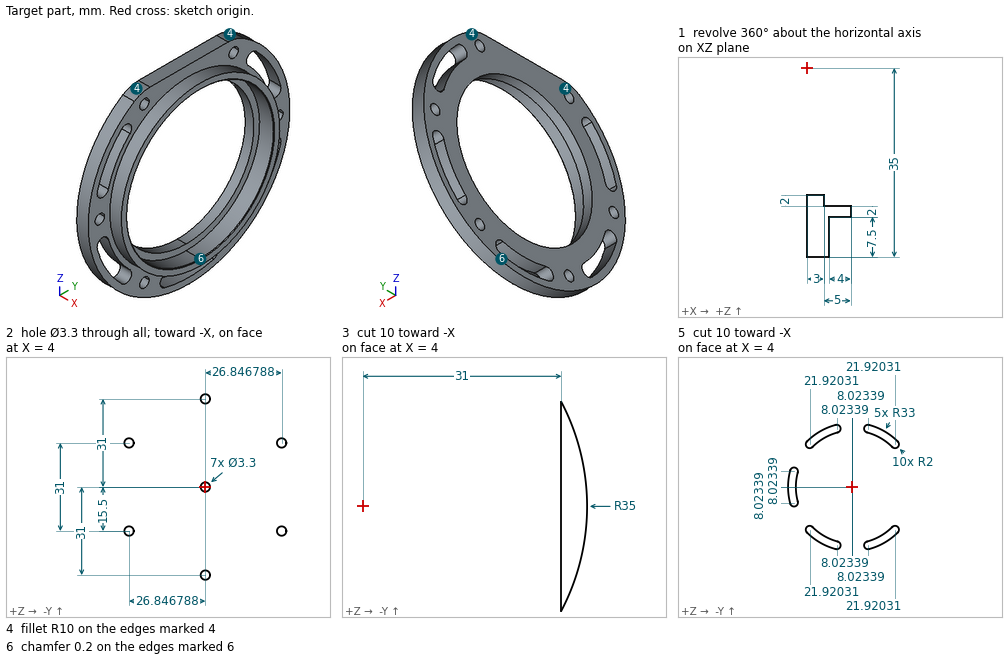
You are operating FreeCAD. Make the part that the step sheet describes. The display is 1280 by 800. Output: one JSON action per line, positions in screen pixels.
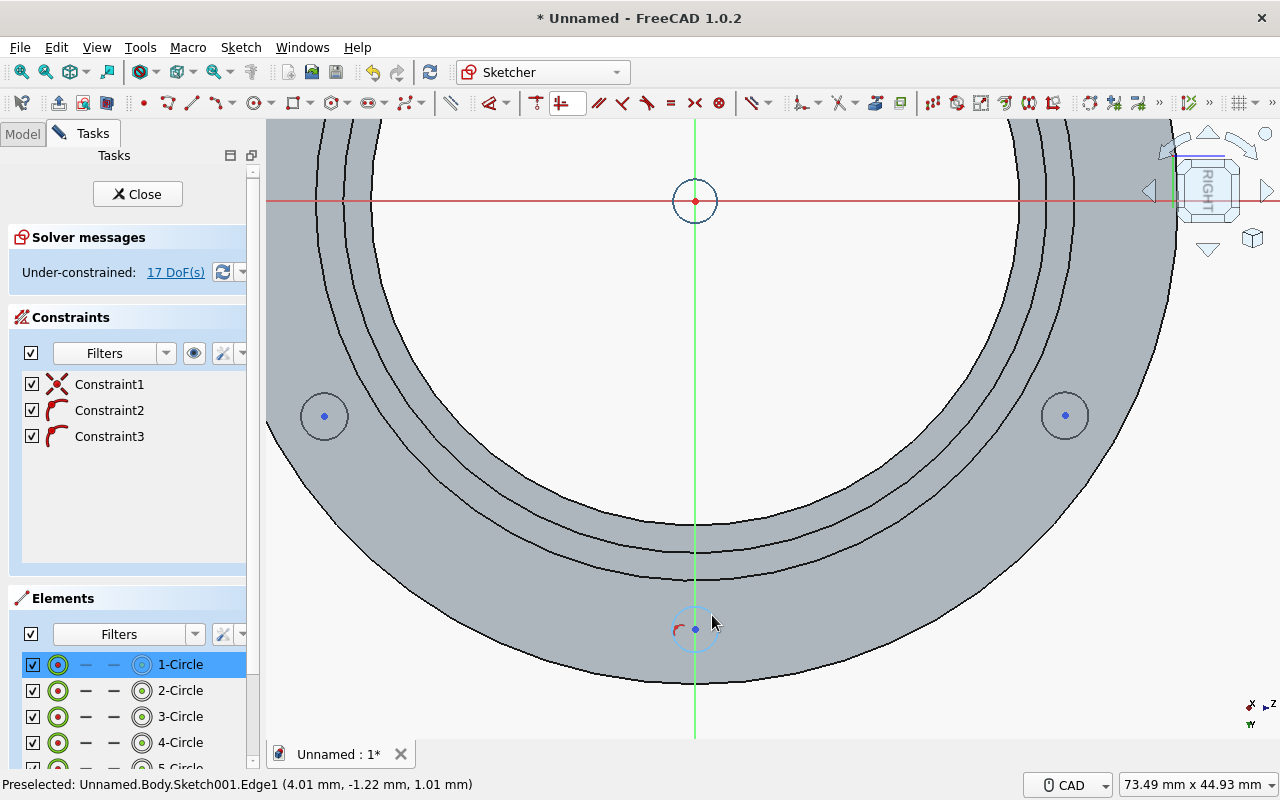
{"action": "left_click", "coordinate": [711, 613]}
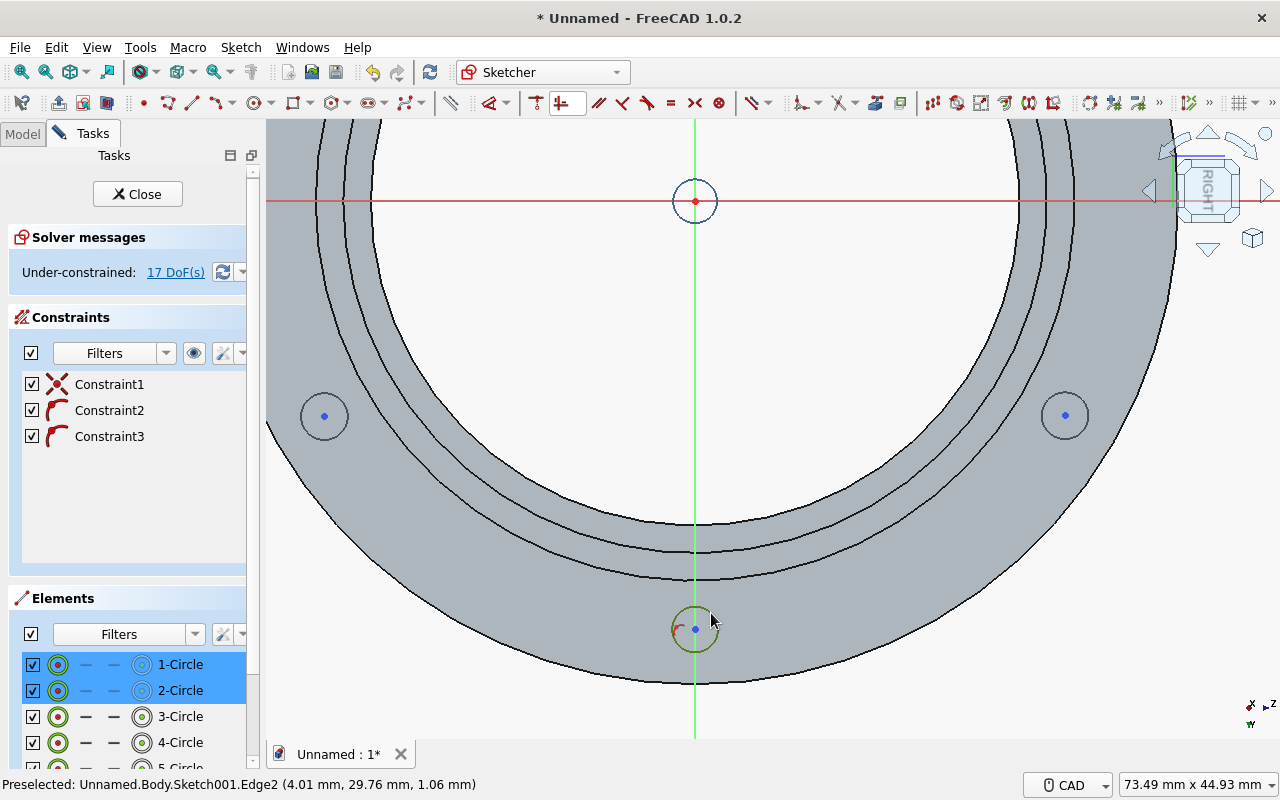
{"action": "left_click", "coordinate": [341, 400]}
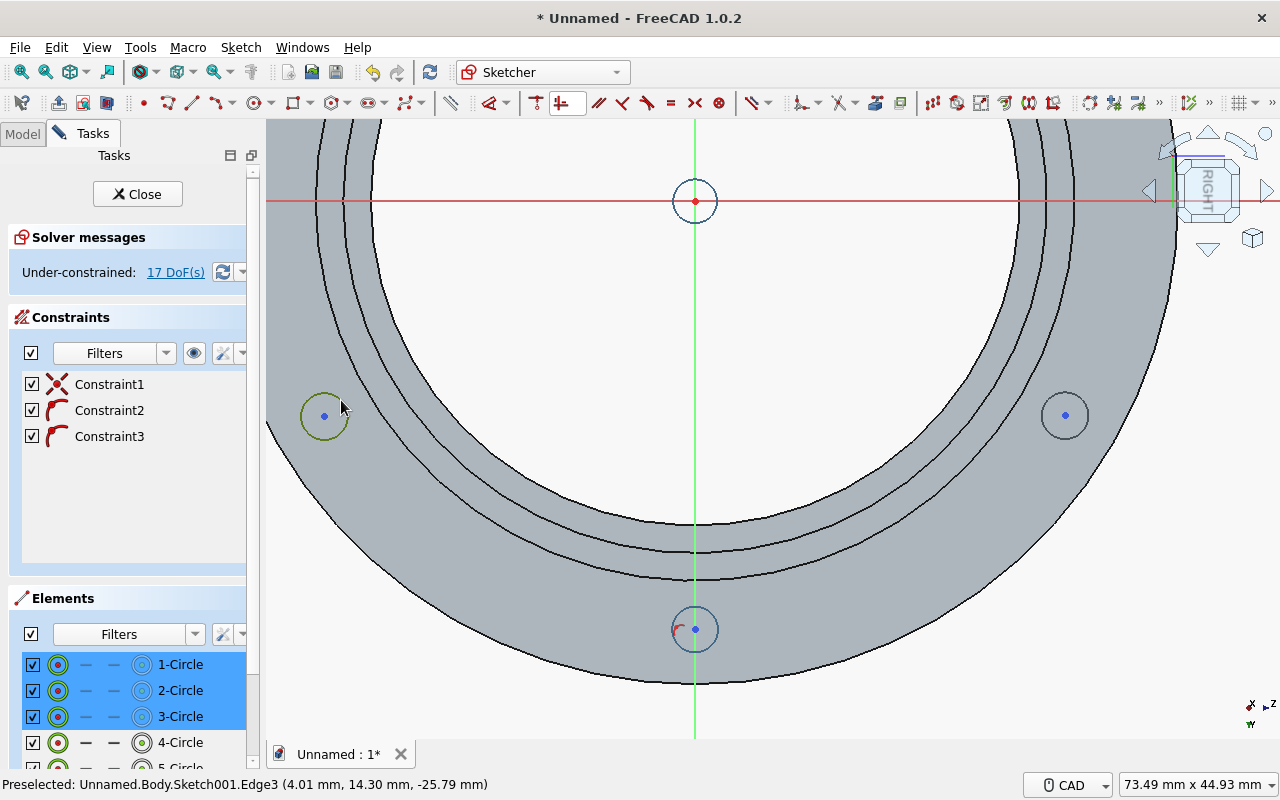
{"action": "scroll", "coordinate": [712, 615], "scroll_direction": "down", "scroll_amount": 4}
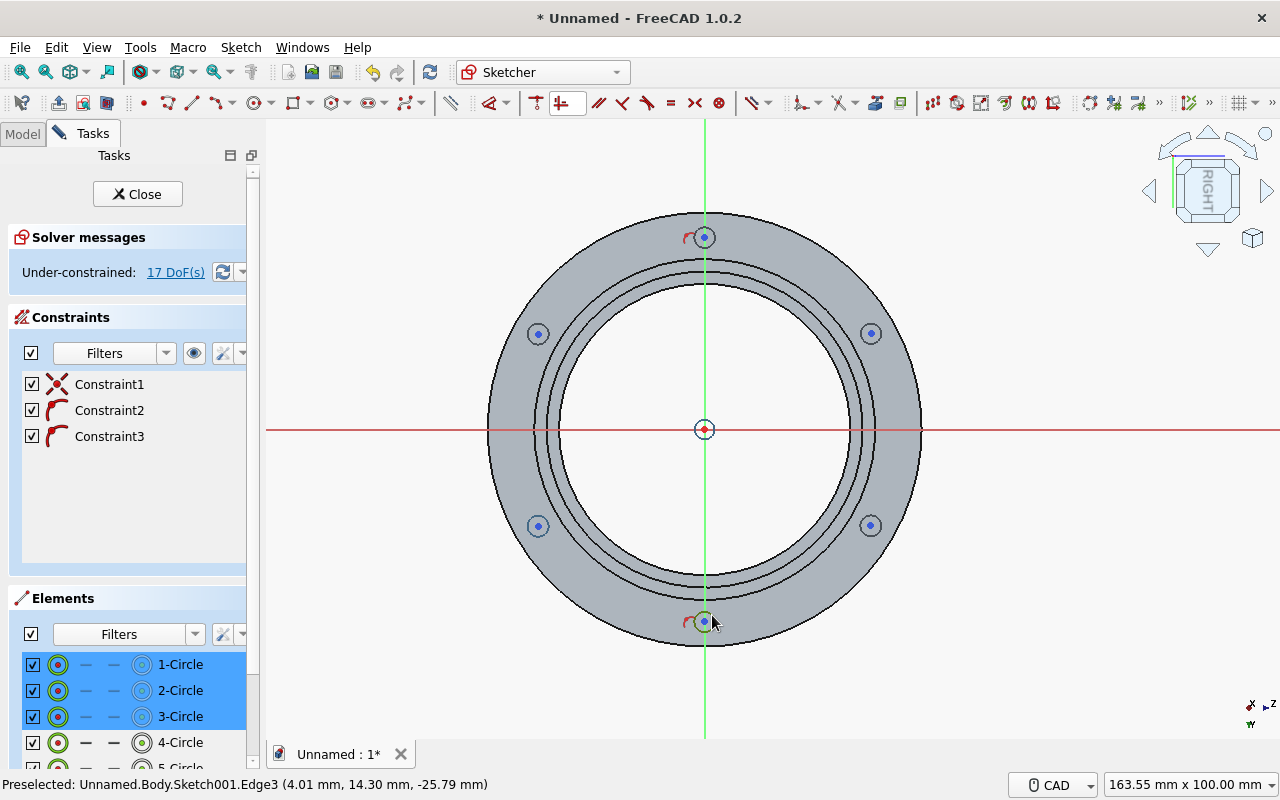
{"action": "scroll", "coordinate": [546, 327], "scroll_direction": "up", "scroll_amount": 2}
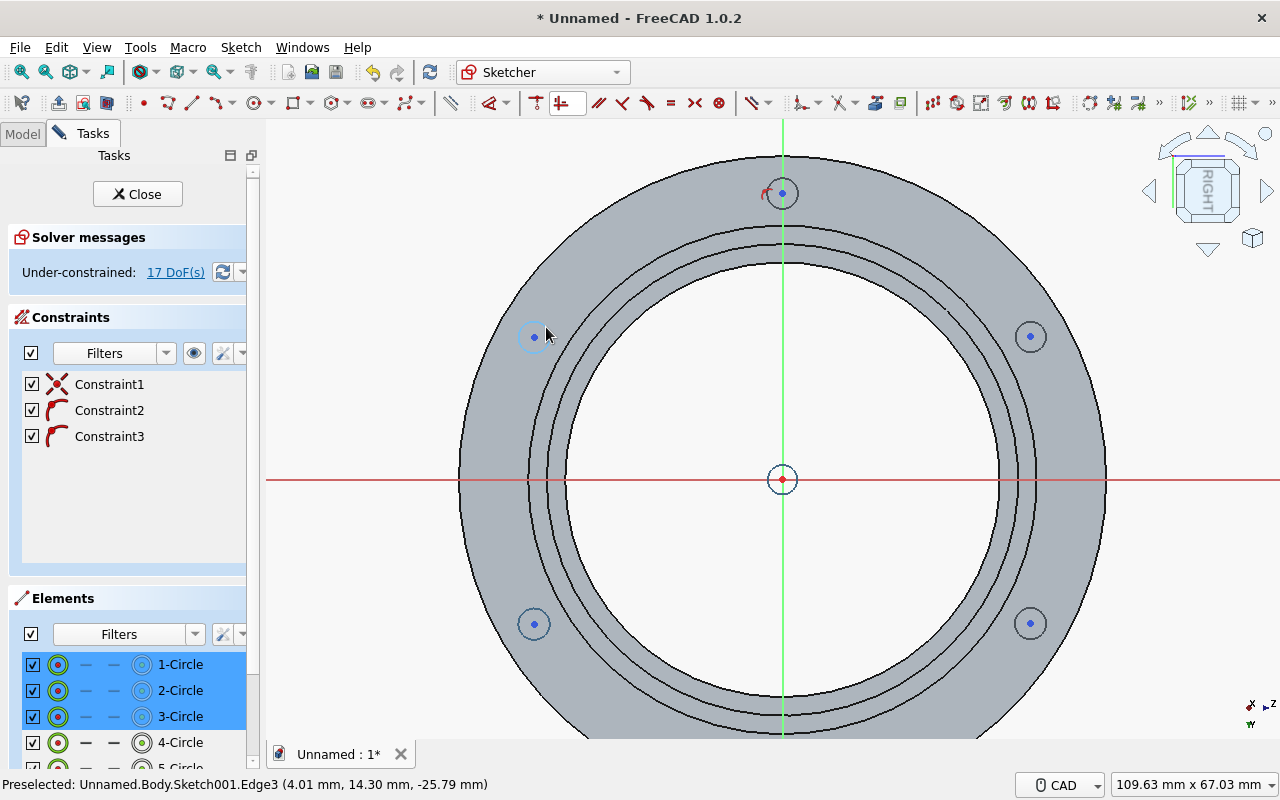
{"action": "left_click", "coordinate": [545, 326]}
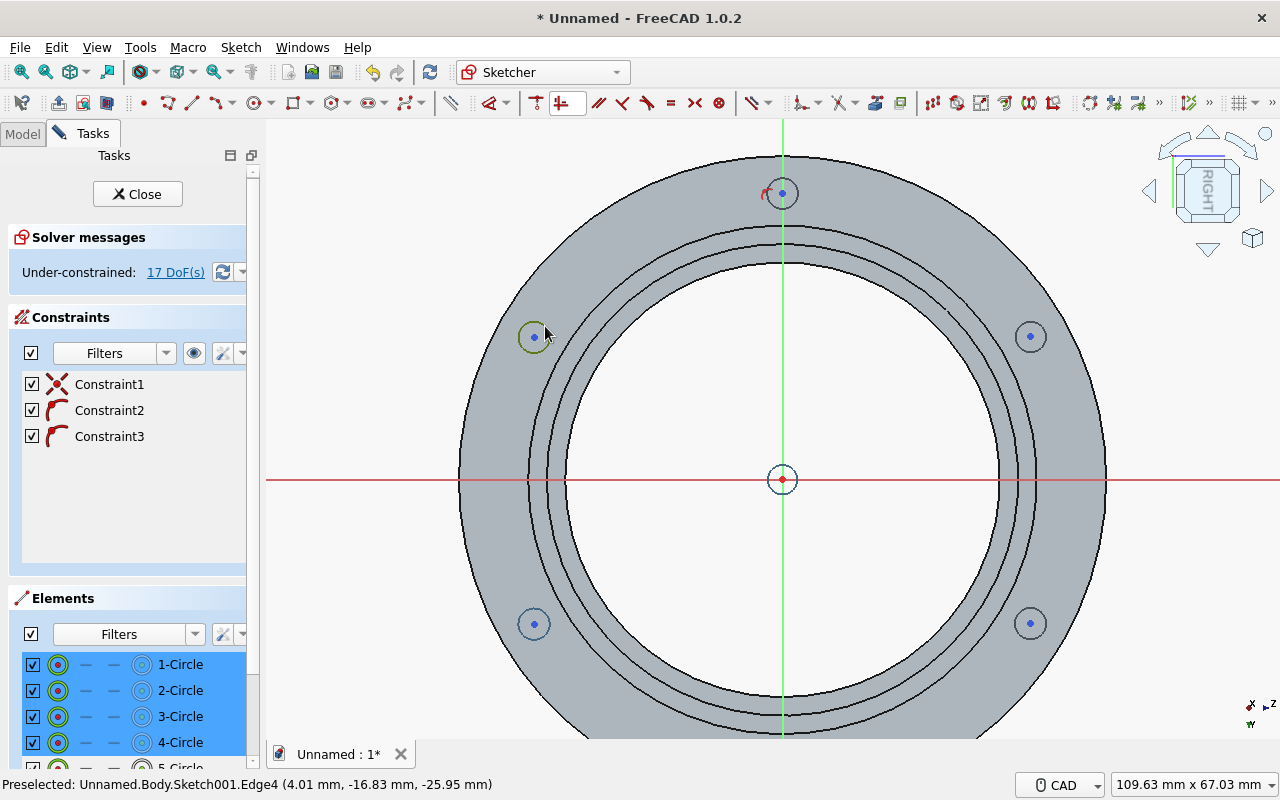
{"action": "scroll", "coordinate": [793, 183], "scroll_direction": "up", "scroll_amount": 2}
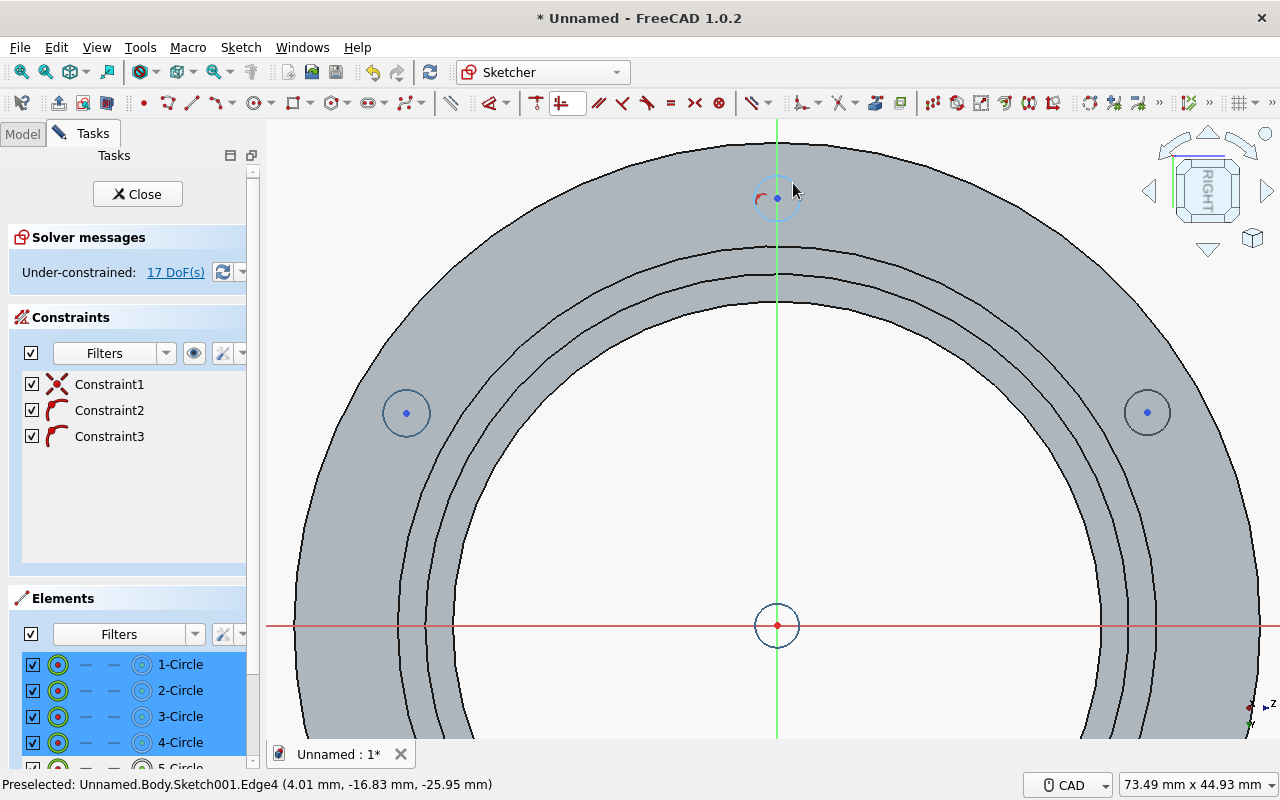
{"action": "left_click", "coordinate": [793, 182]}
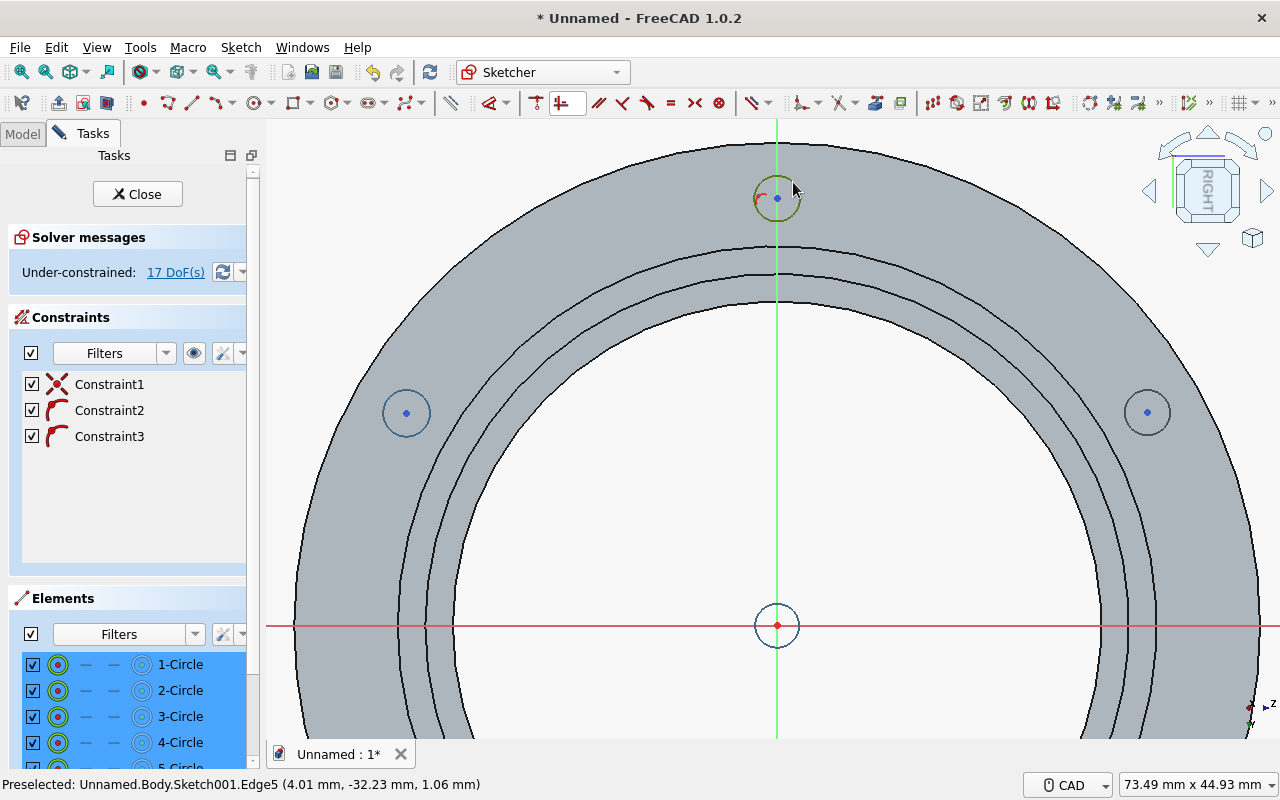
{"action": "scroll", "coordinate": [645, 268], "scroll_direction": "down", "scroll_amount": 4}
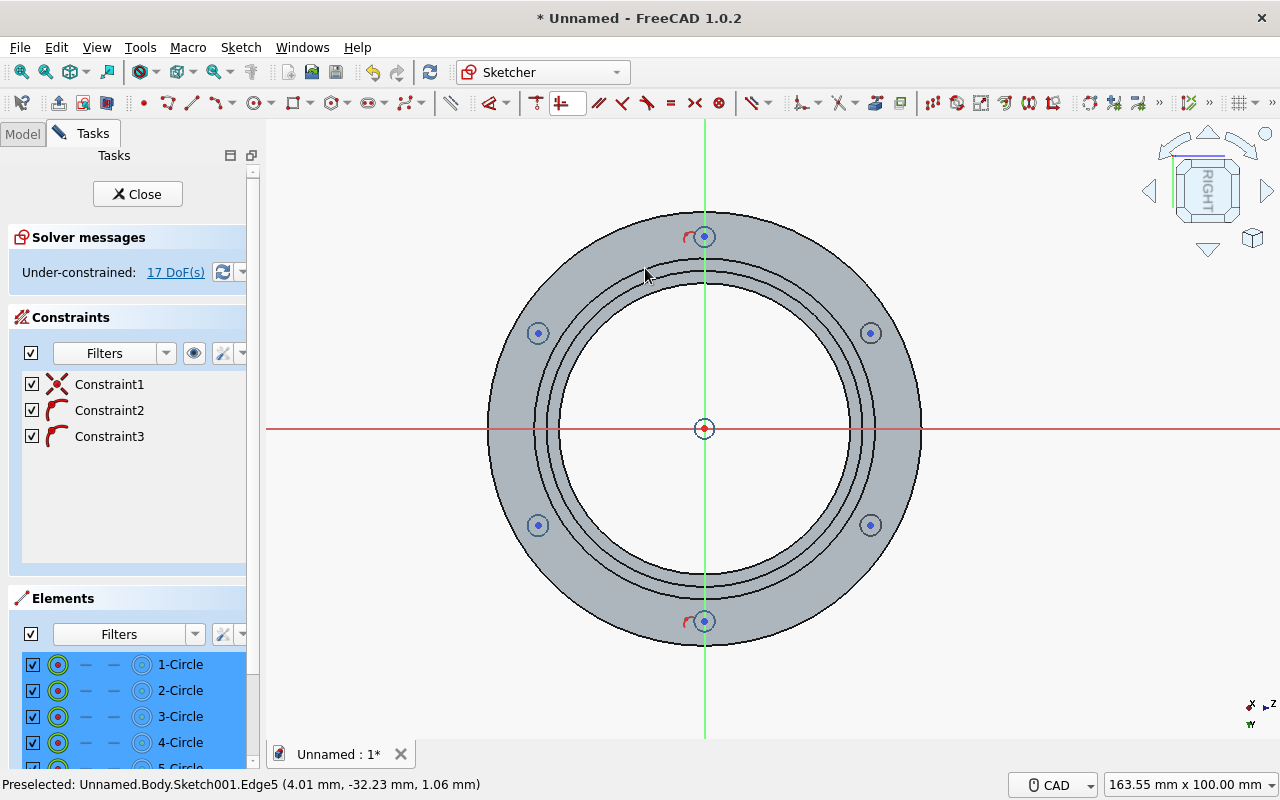
{"action": "scroll", "coordinate": [878, 326], "scroll_direction": "up", "scroll_amount": 2}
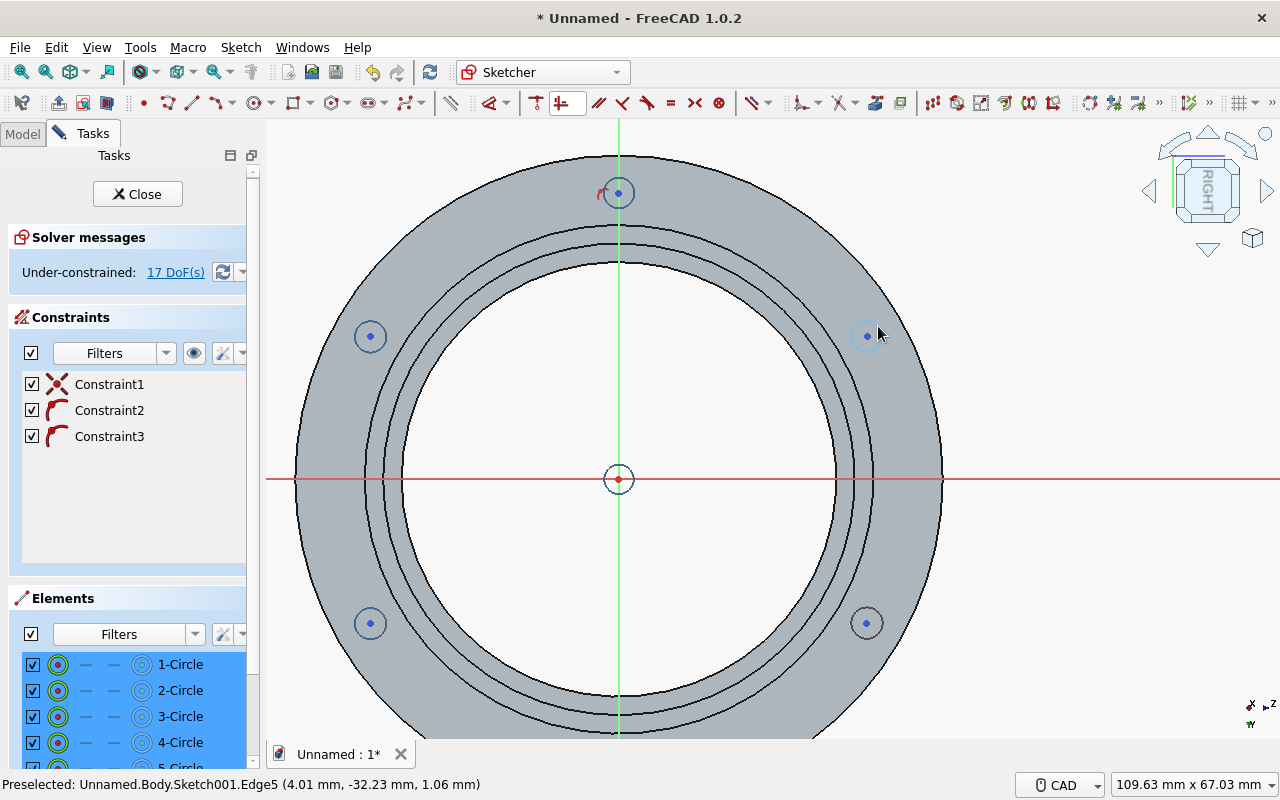
{"action": "left_click", "coordinate": [878, 326]}